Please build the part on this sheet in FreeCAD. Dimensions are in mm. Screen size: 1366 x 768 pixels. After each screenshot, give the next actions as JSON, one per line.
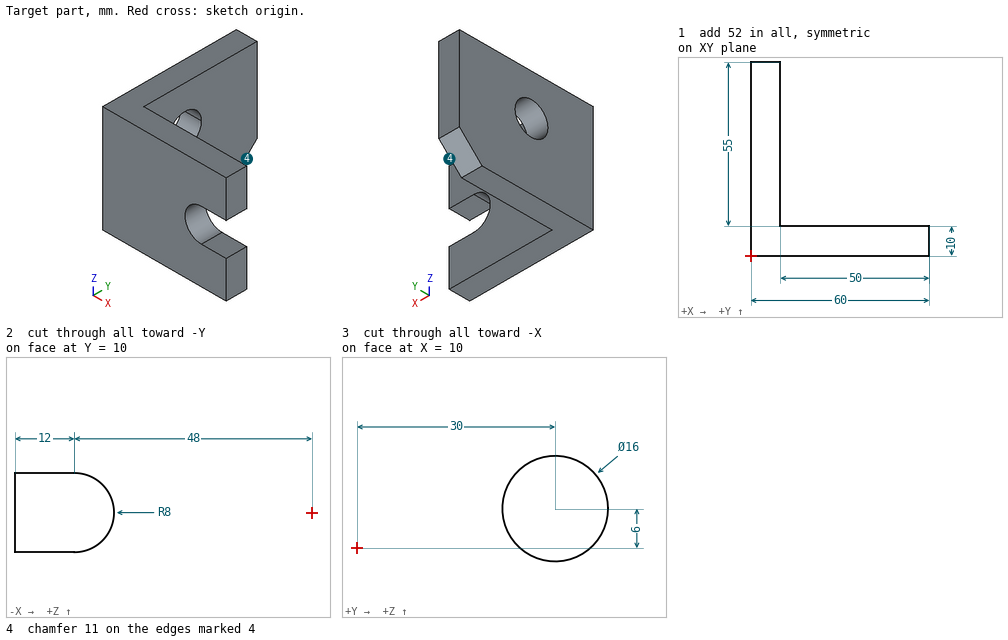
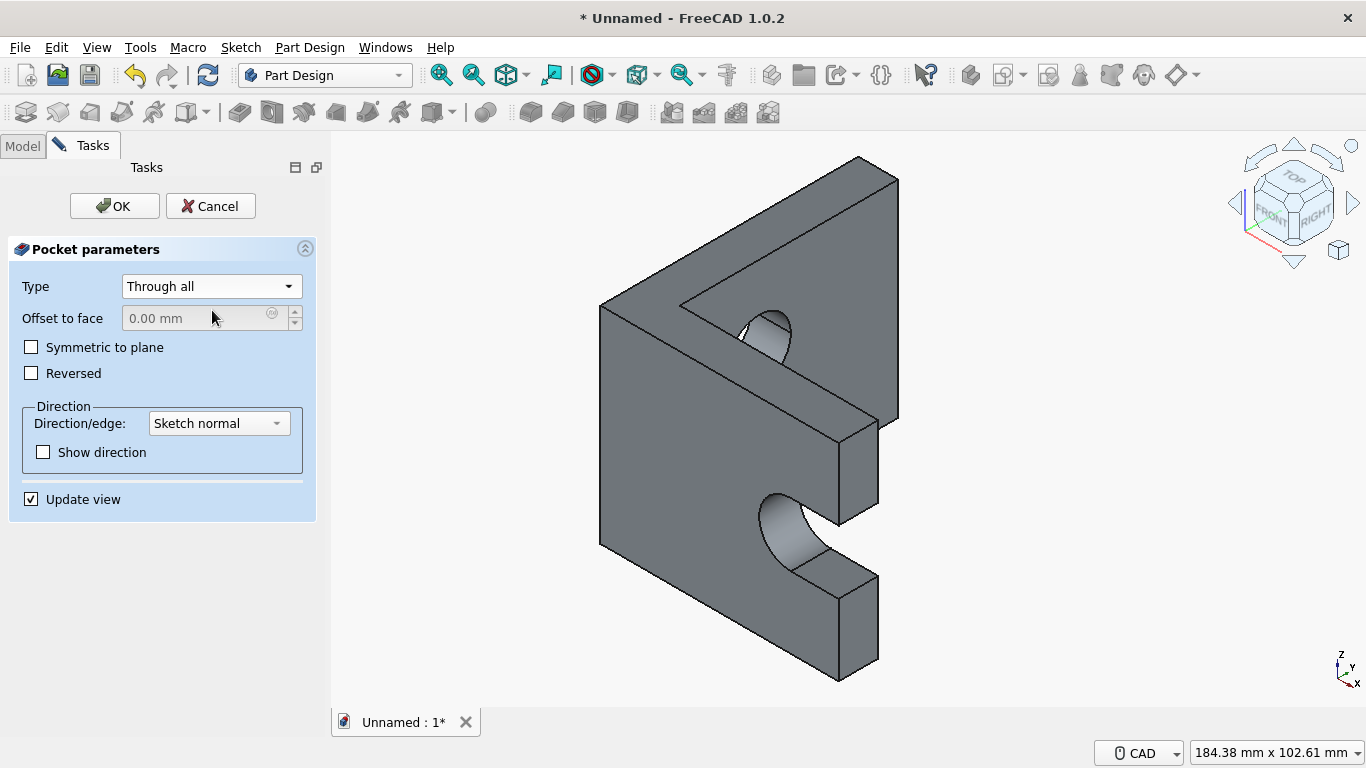
{"action": "left_click", "coordinate": [115, 206]}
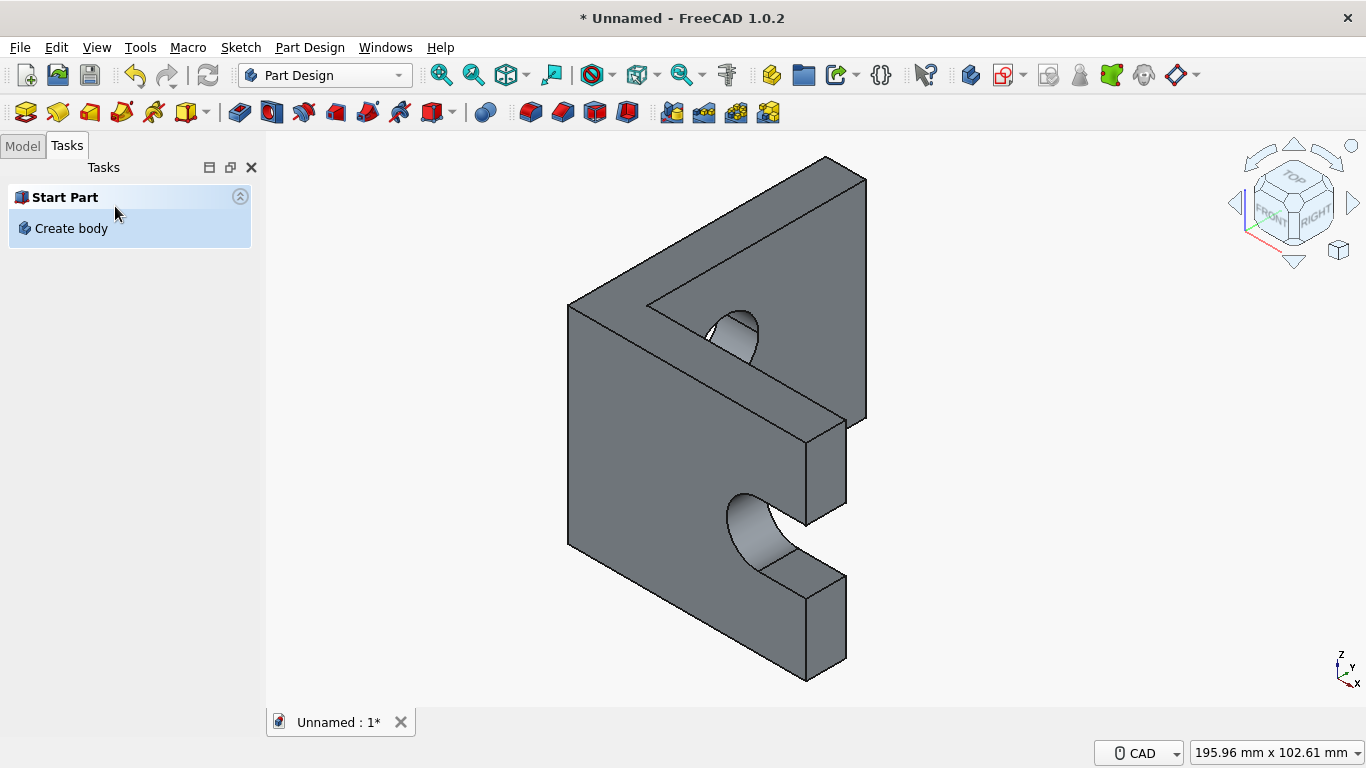
{"action": "key", "text": "2"}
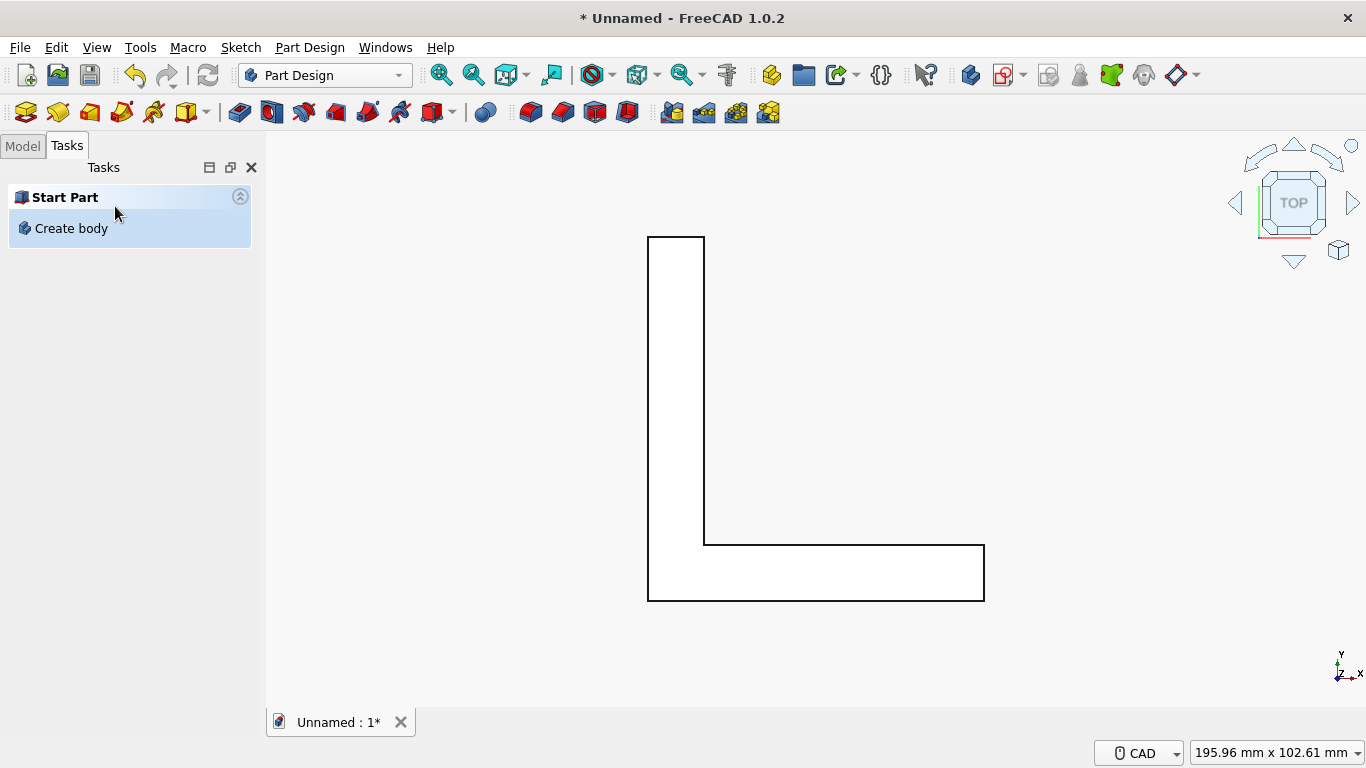
{"action": "key", "text": "0"}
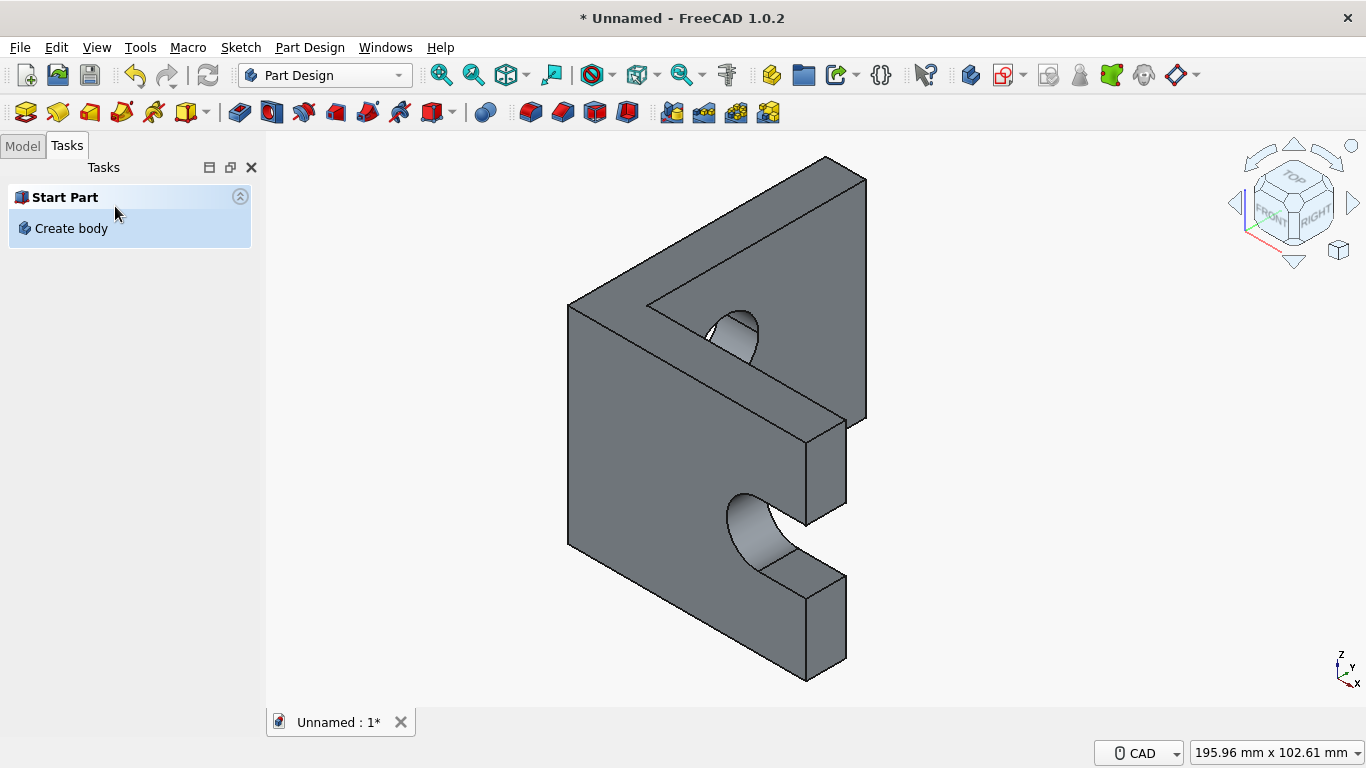
{"action": "key", "text": "1"}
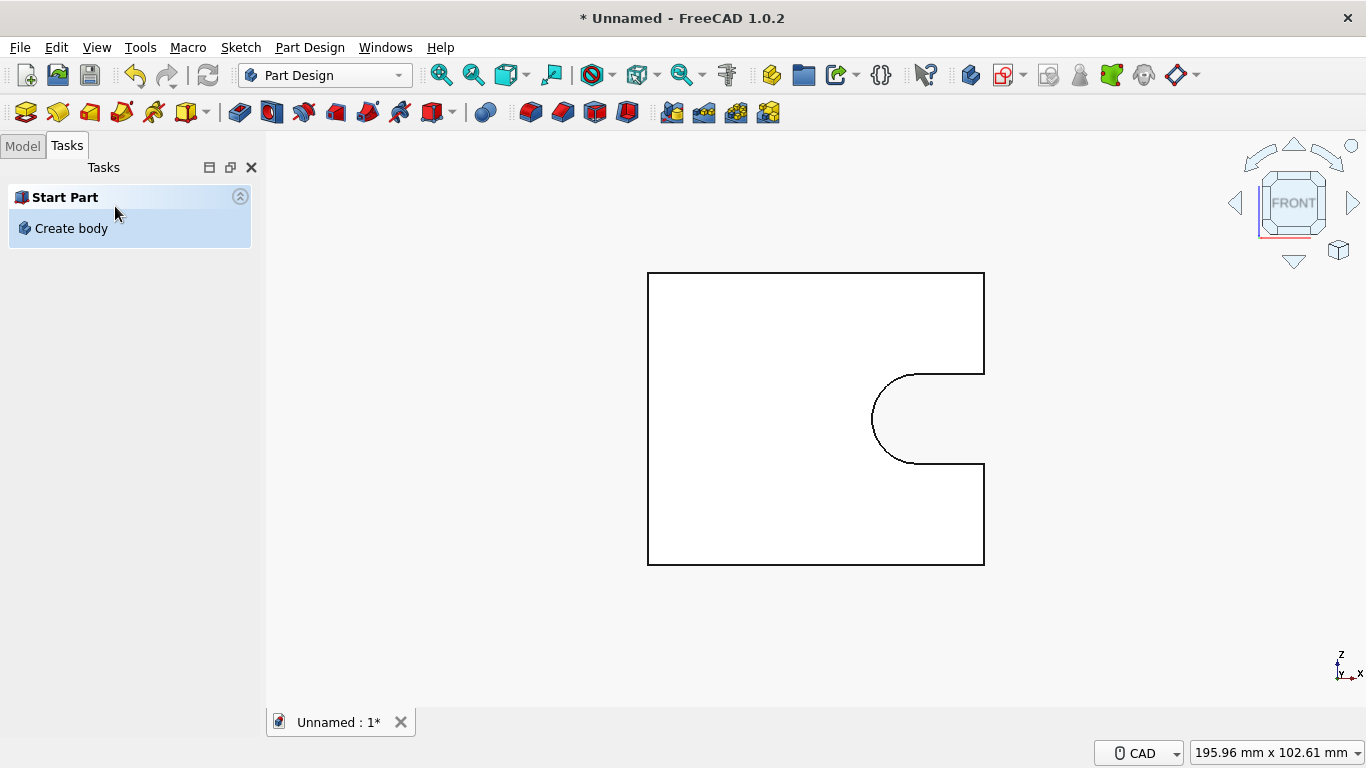
{"action": "key", "text": "3"}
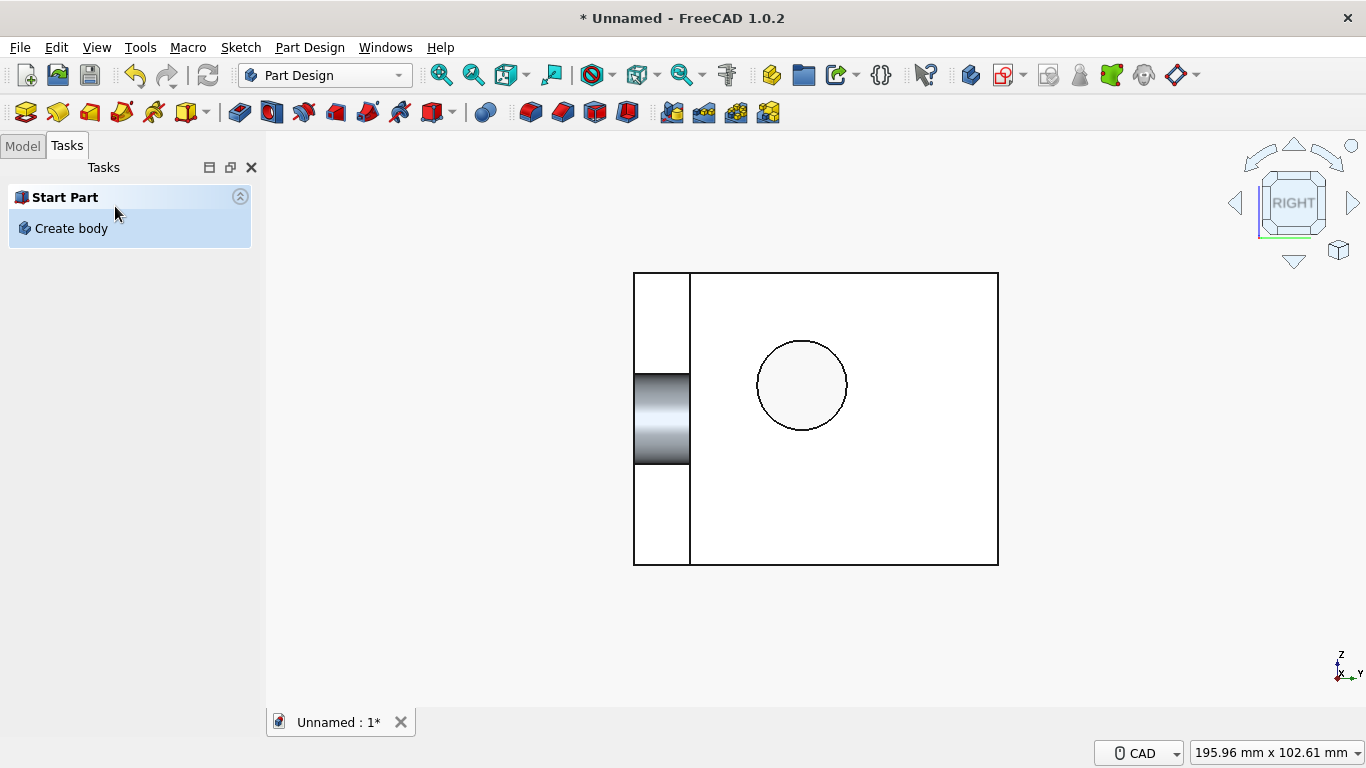
{"action": "key", "text": "5"}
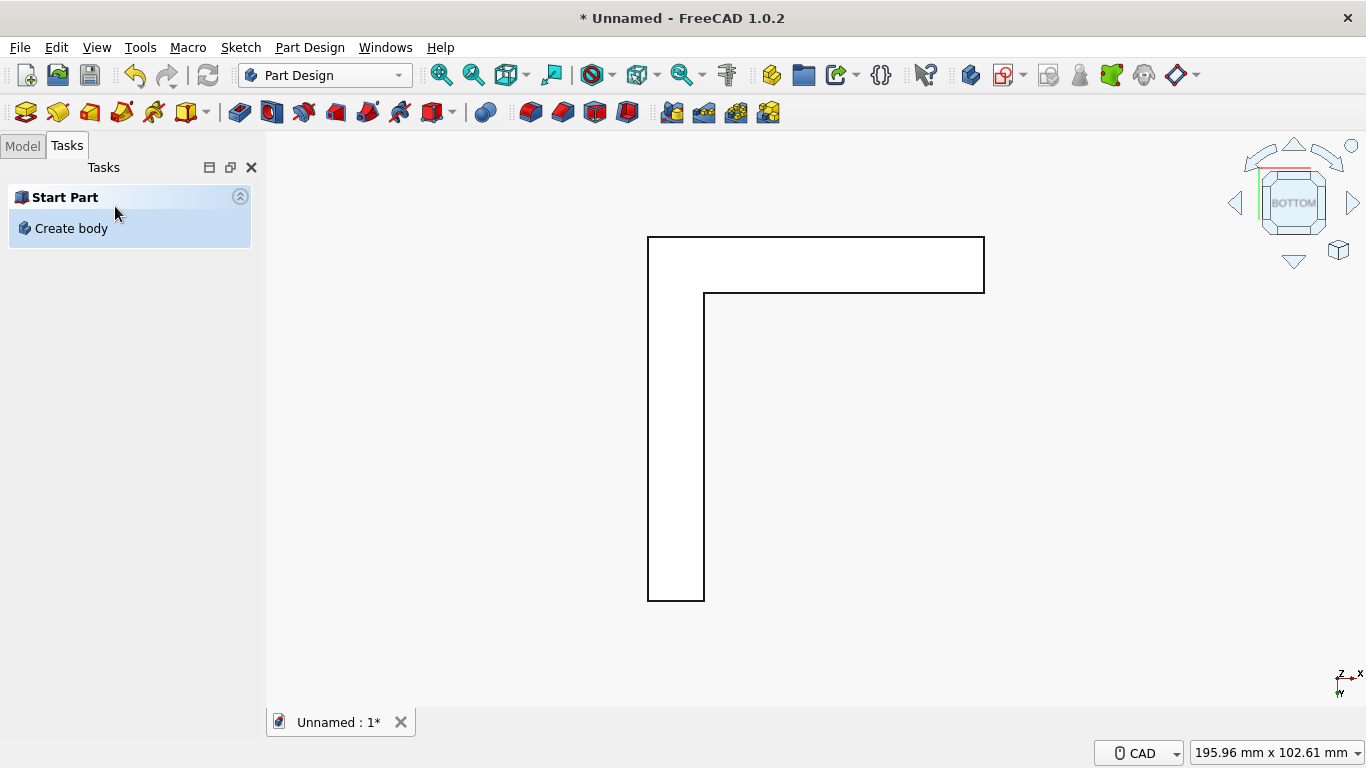
{"action": "left_click", "coordinate": [676, 600]}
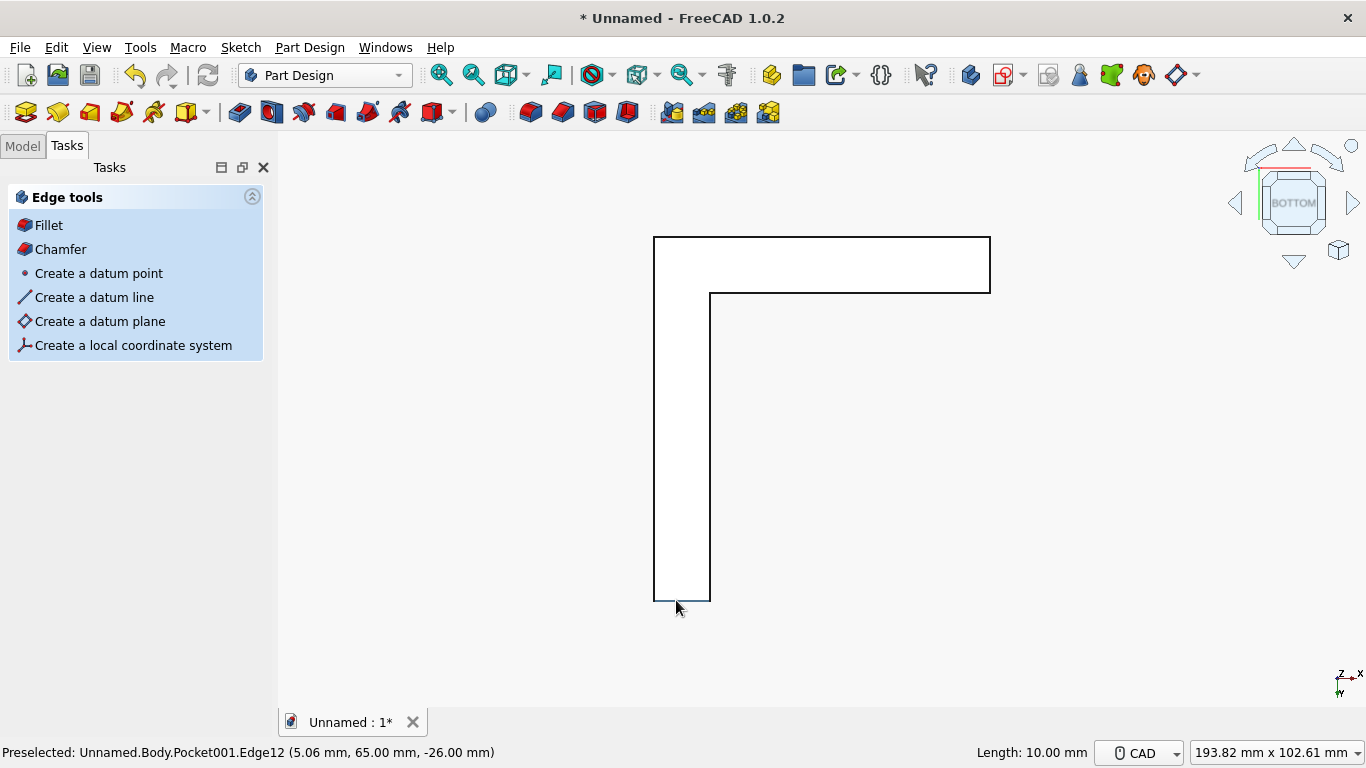
{"action": "left_click", "coordinate": [564, 112]}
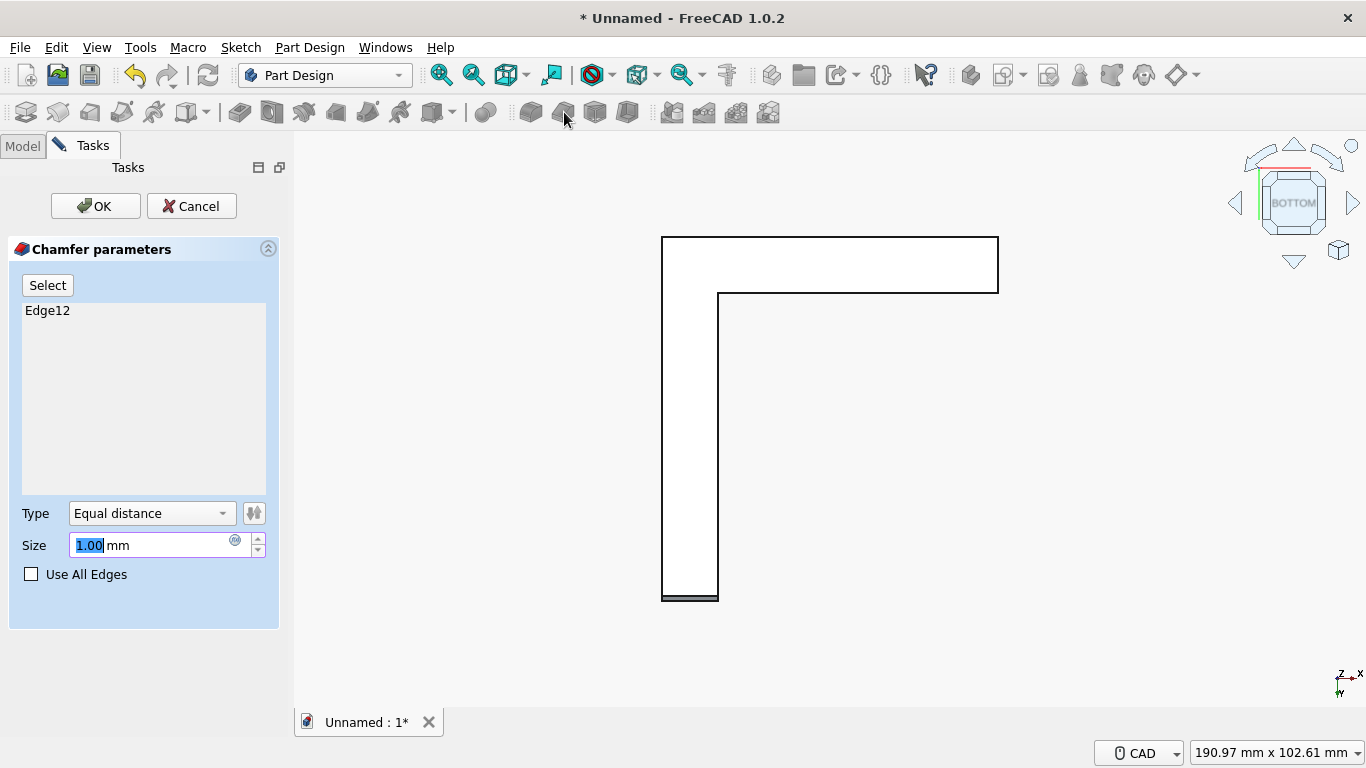
{"action": "type", "text": "11"}
{"action": "key", "text": "Tab"}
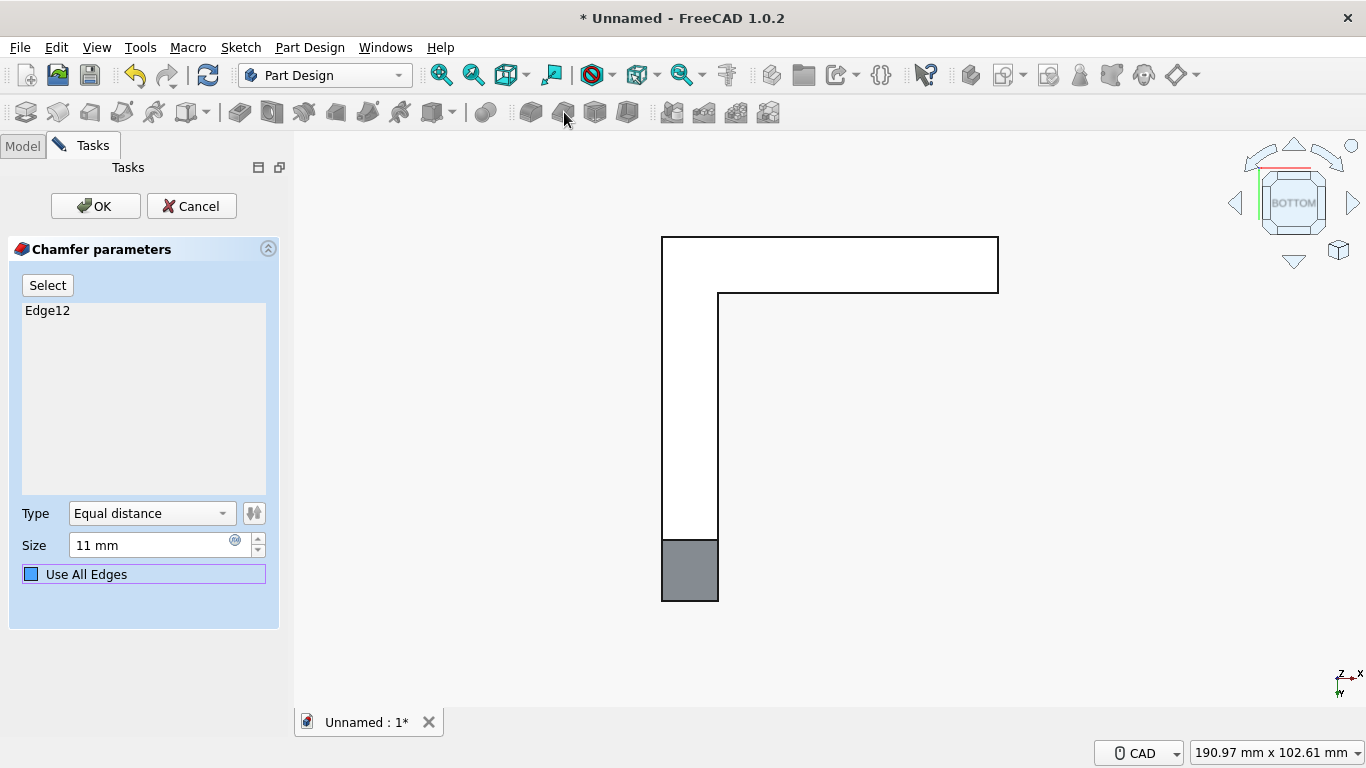
{"action": "left_click", "coordinate": [96, 206]}